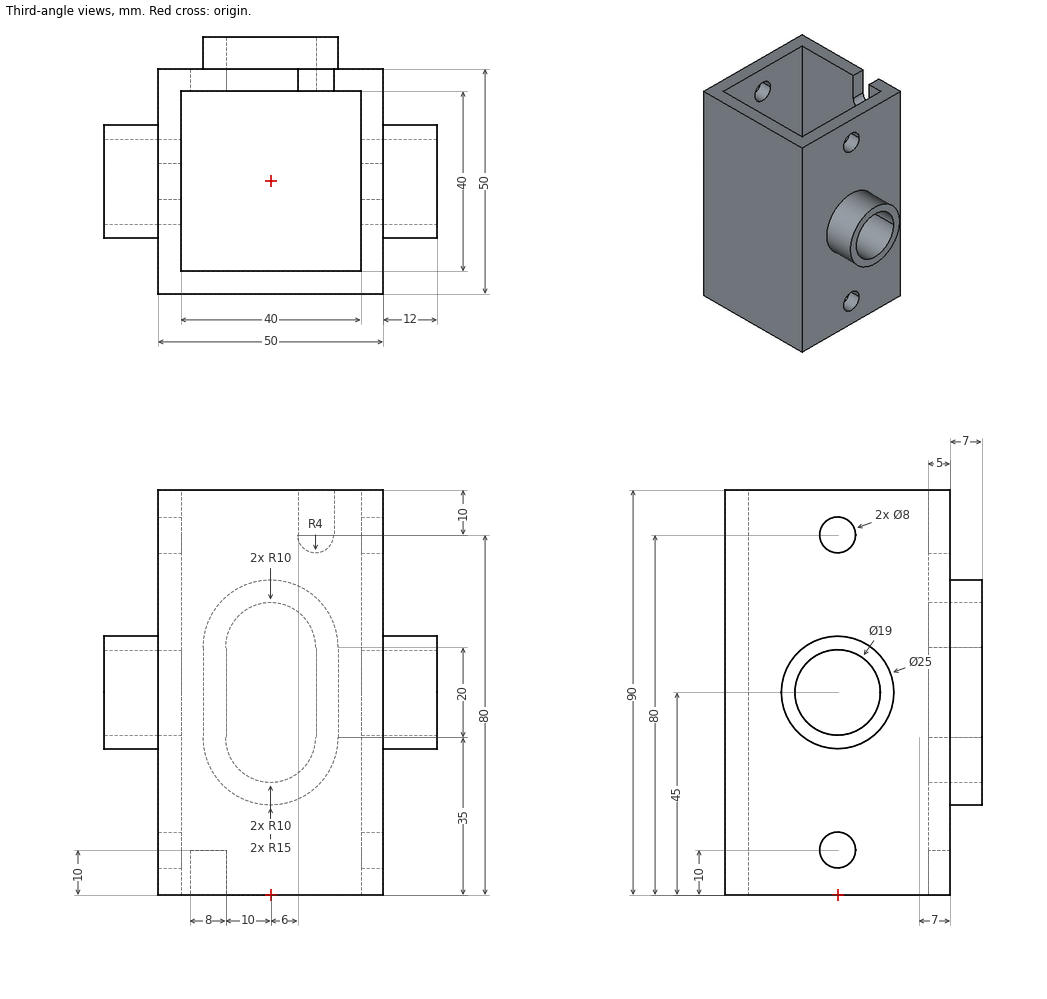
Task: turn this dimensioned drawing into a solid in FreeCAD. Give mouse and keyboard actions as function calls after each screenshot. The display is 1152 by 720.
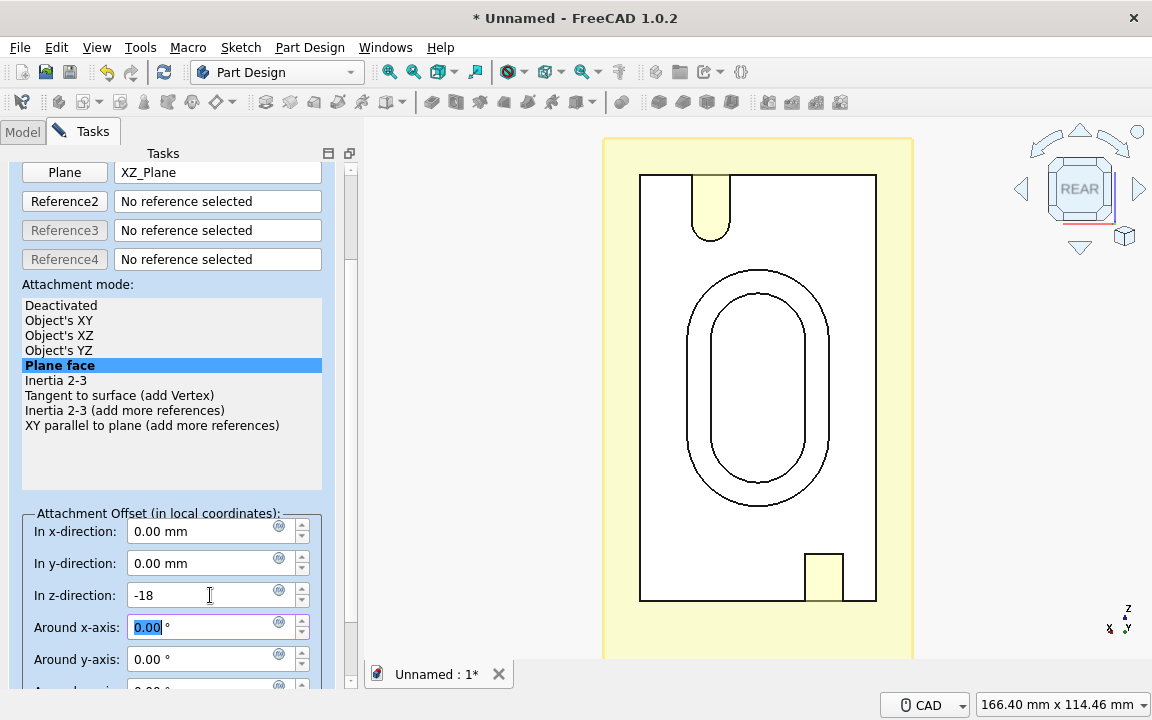
scroll(351, 426, up, 3)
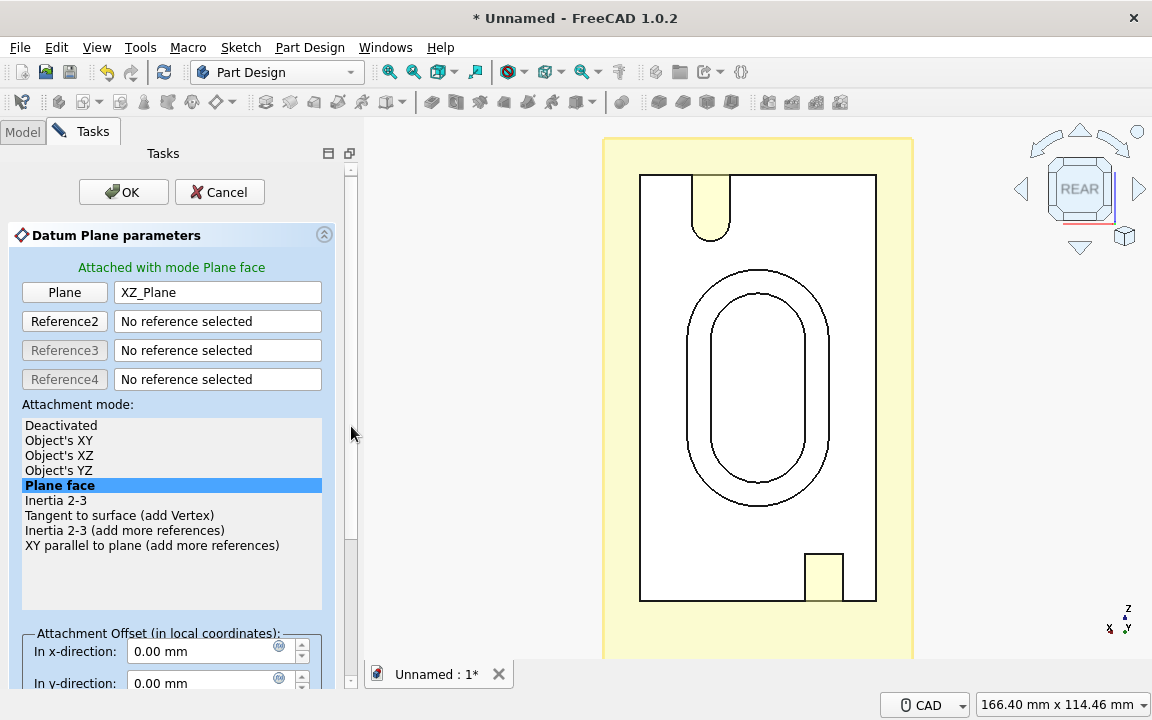
click(124, 192)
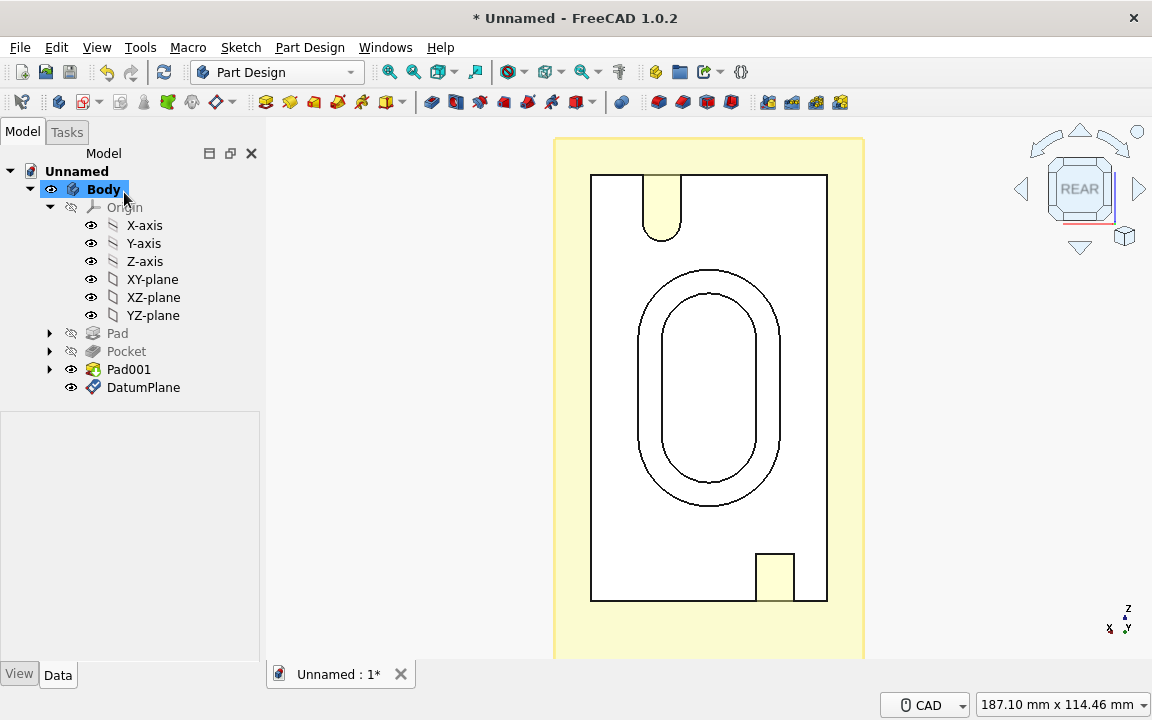
click(116, 387)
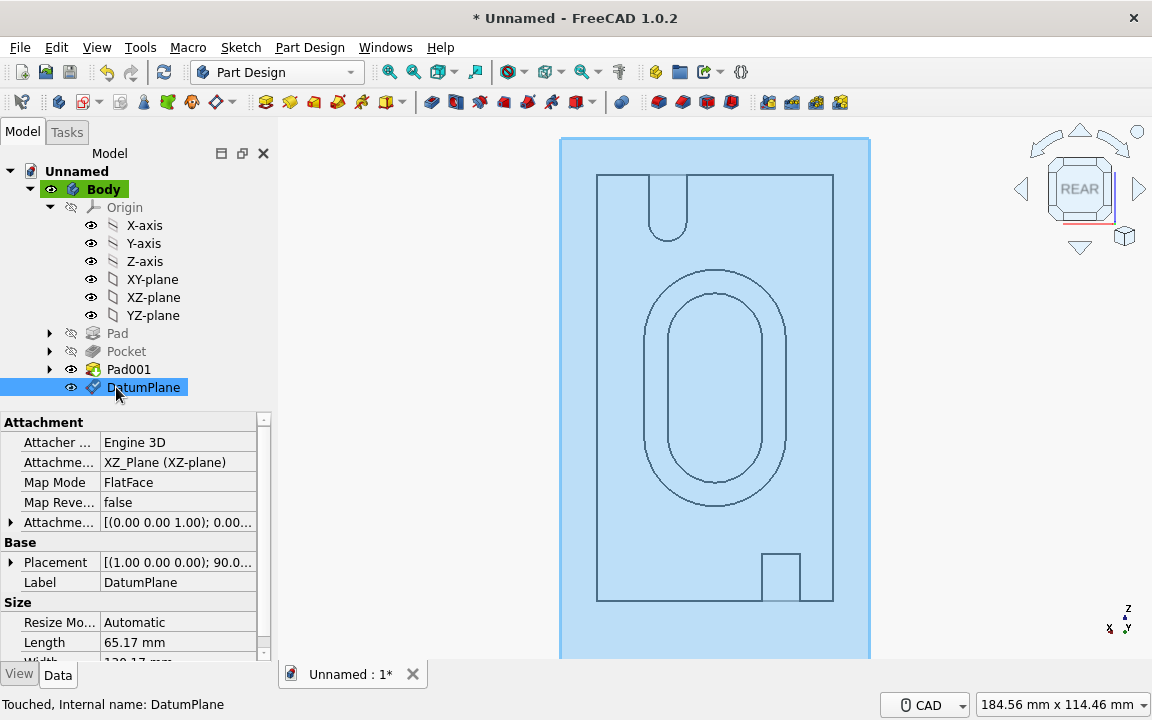
click(84, 102)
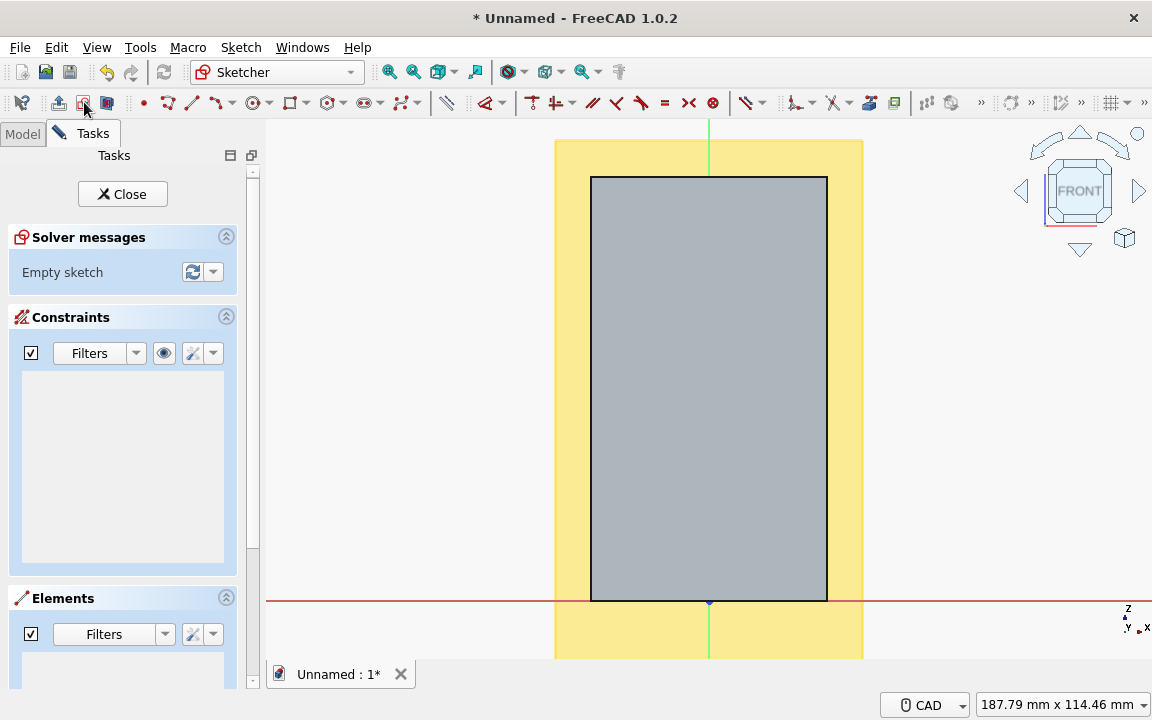
key(q)
key(s)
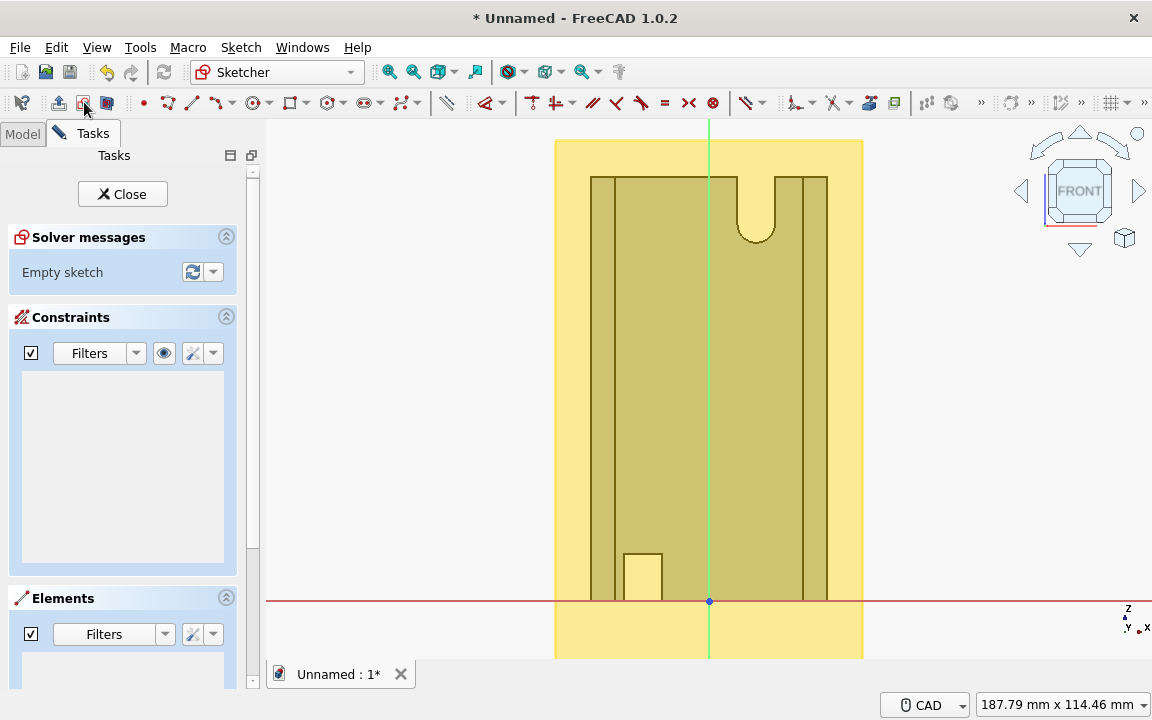
key(g)
key(s)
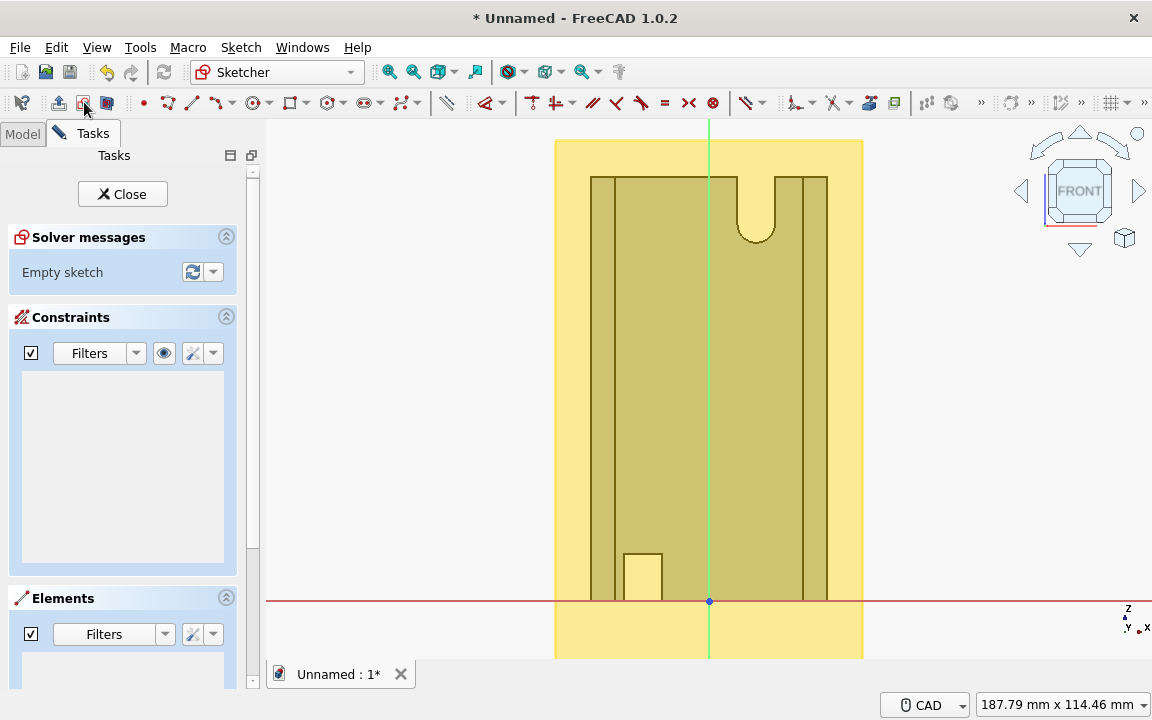
click(709, 436)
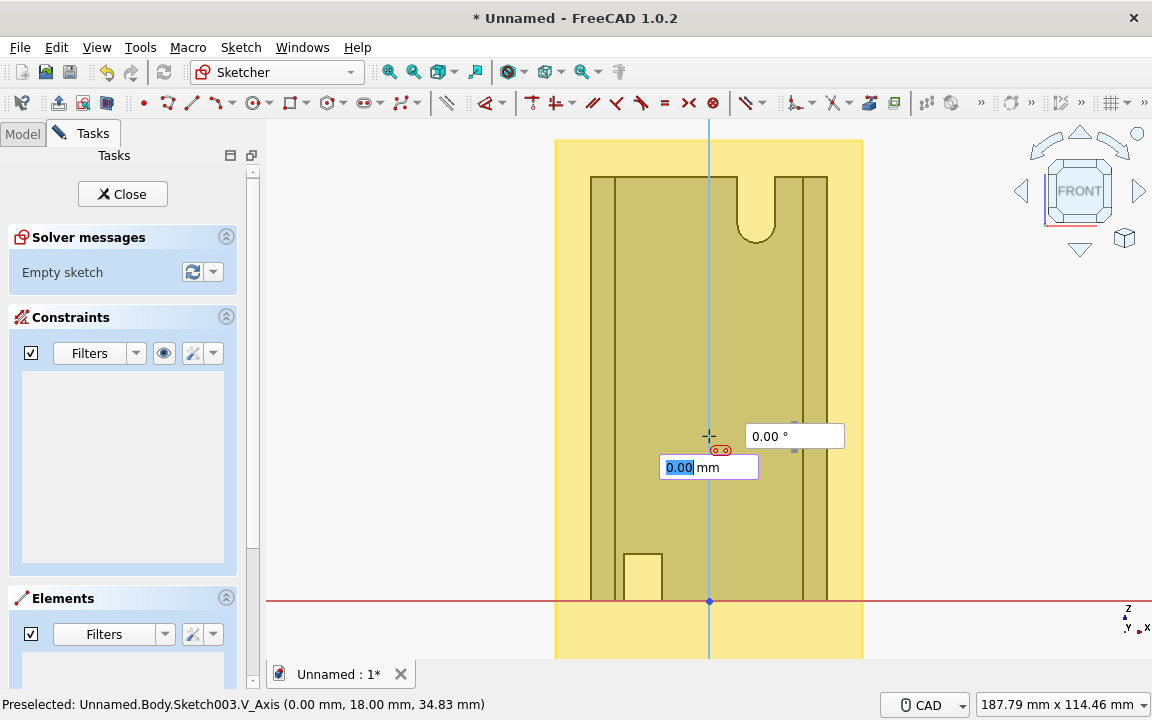
click(718, 342)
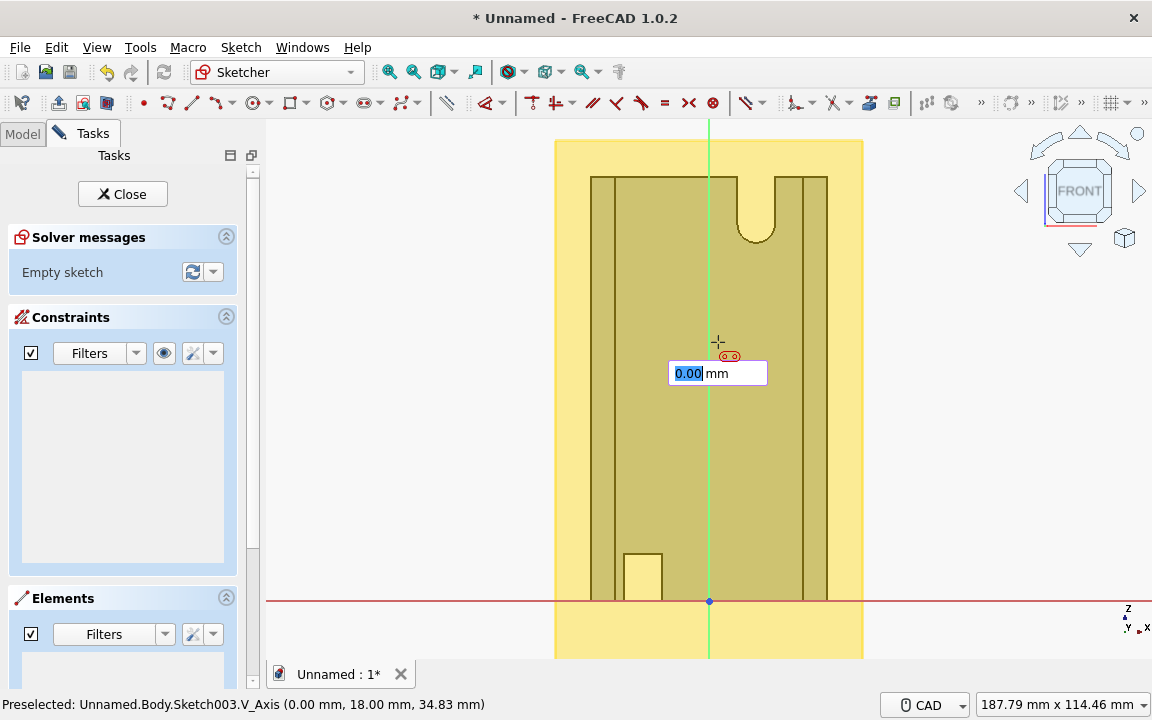
click(756, 389)
key(Escape)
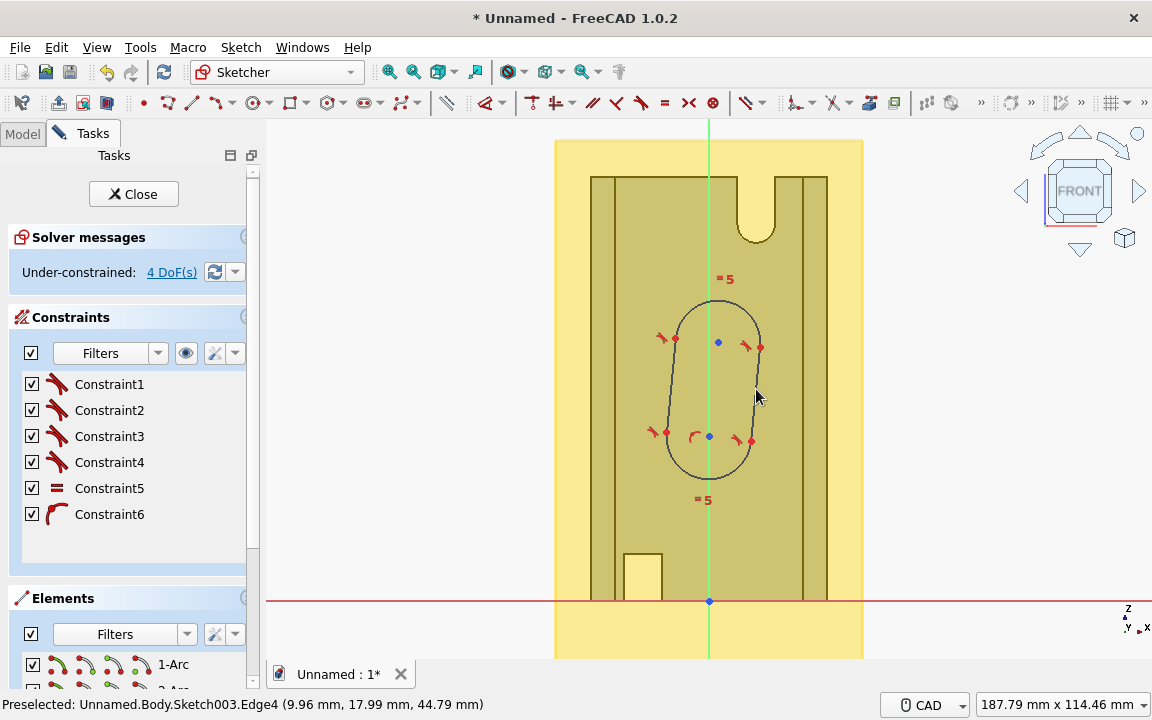
click(670, 405)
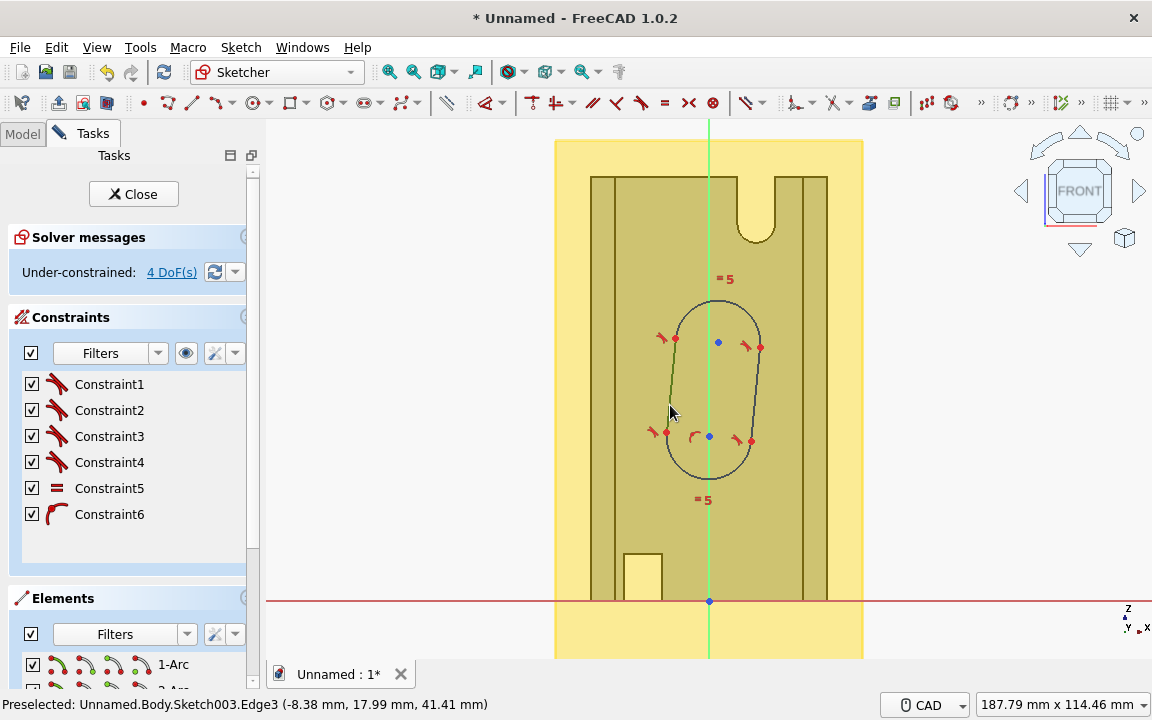
click(574, 104)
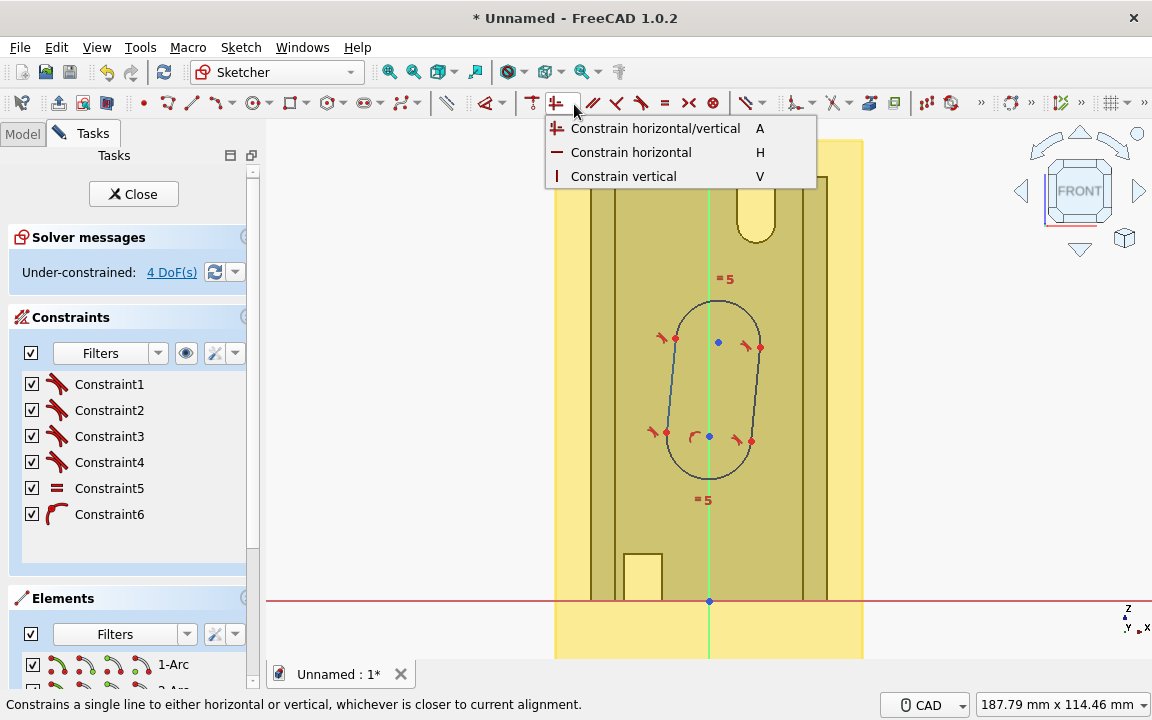
click(681, 176)